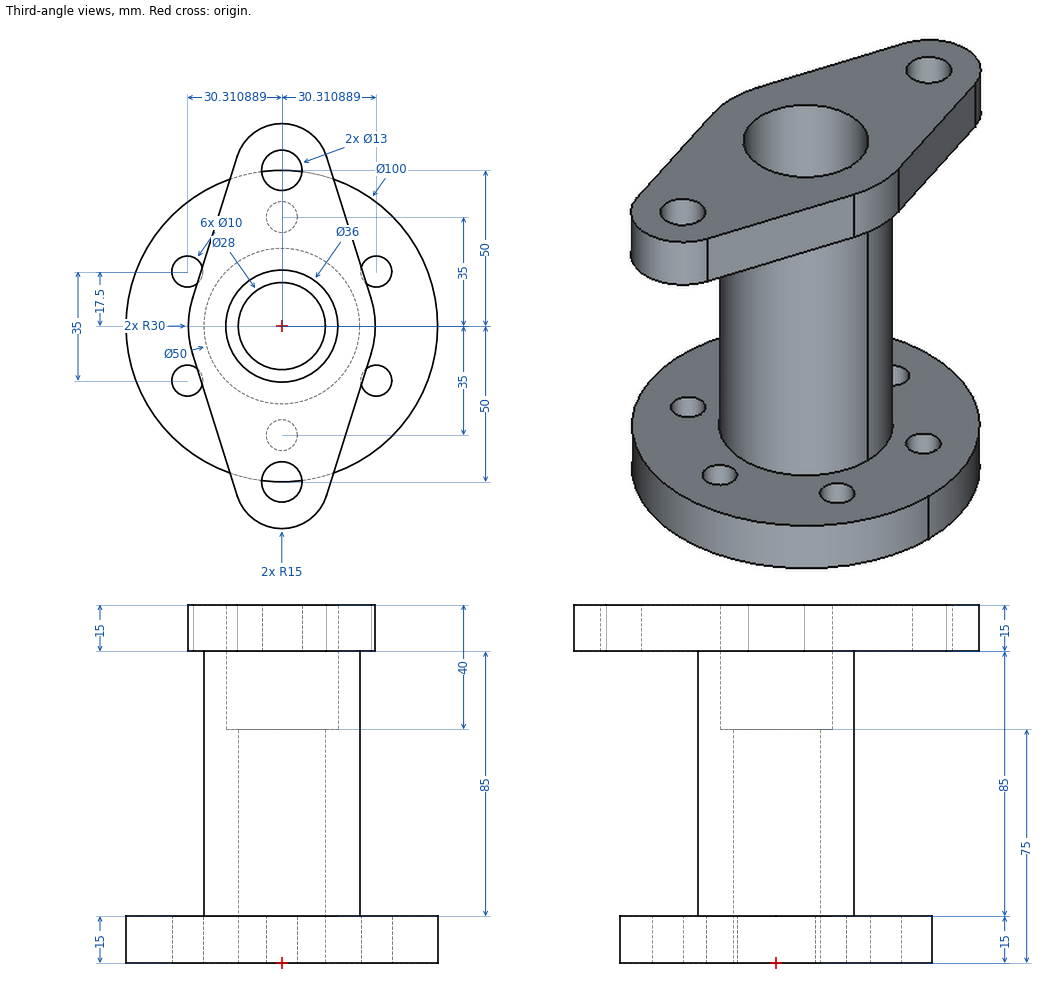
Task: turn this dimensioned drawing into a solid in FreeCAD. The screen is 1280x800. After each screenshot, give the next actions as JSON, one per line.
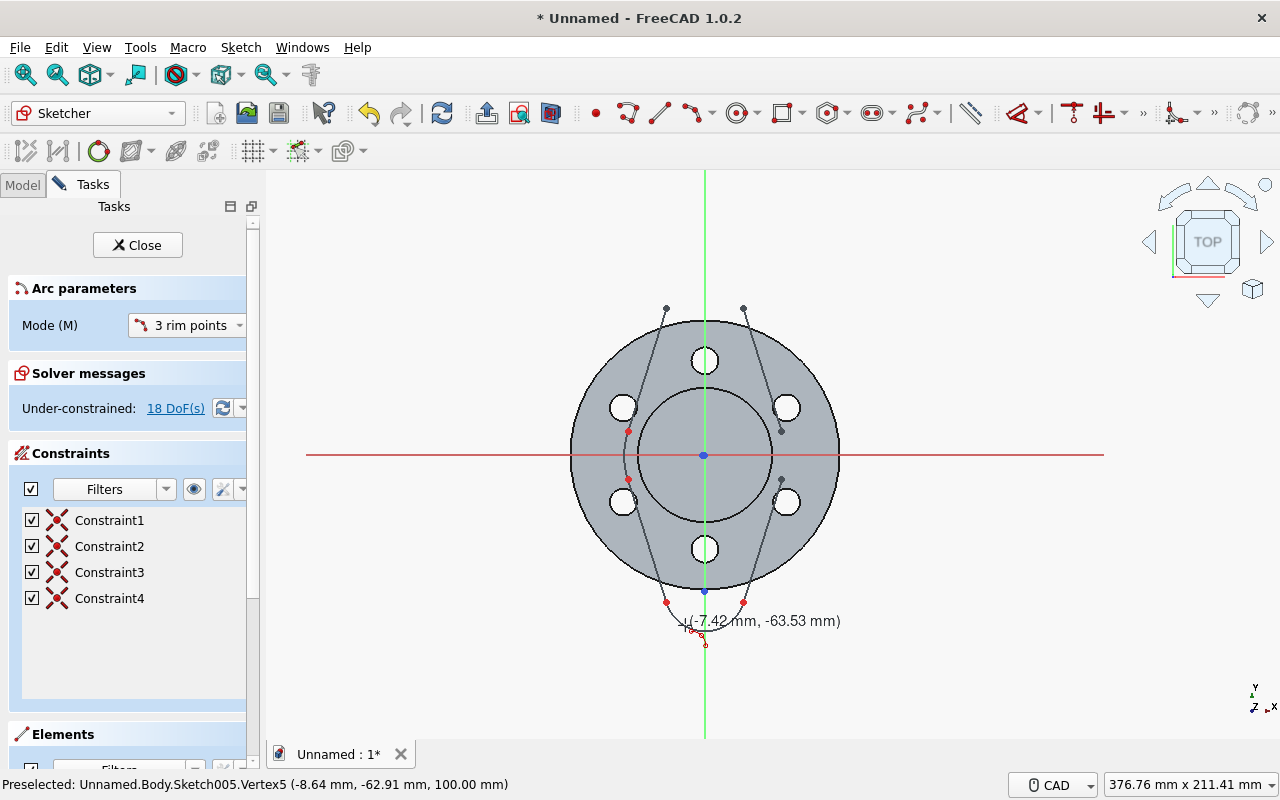
{"action": "left_click", "coordinate": [782, 480]}
{"action": "left_click", "coordinate": [782, 432]}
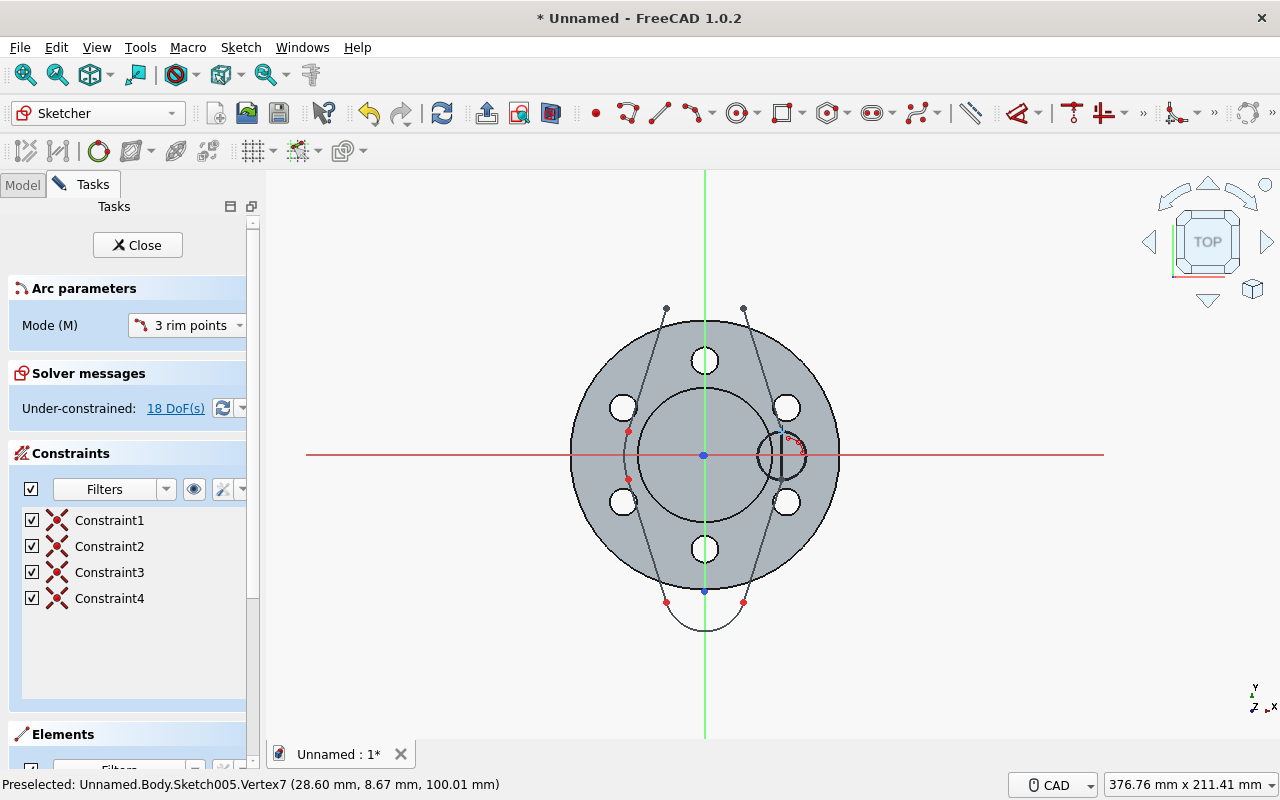
{"action": "scroll", "coordinate": [786, 460], "scroll_direction": "up", "scroll_amount": 8}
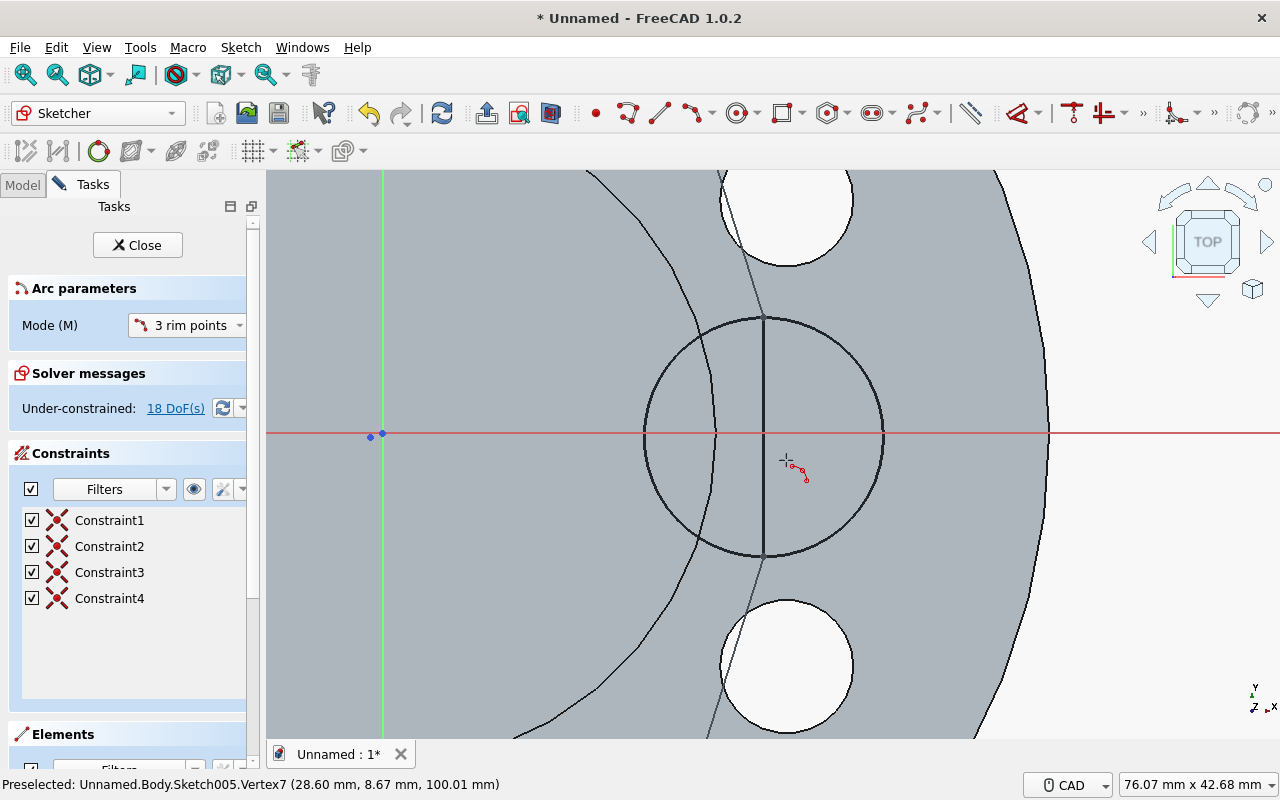
{"action": "left_click", "coordinate": [782, 458]}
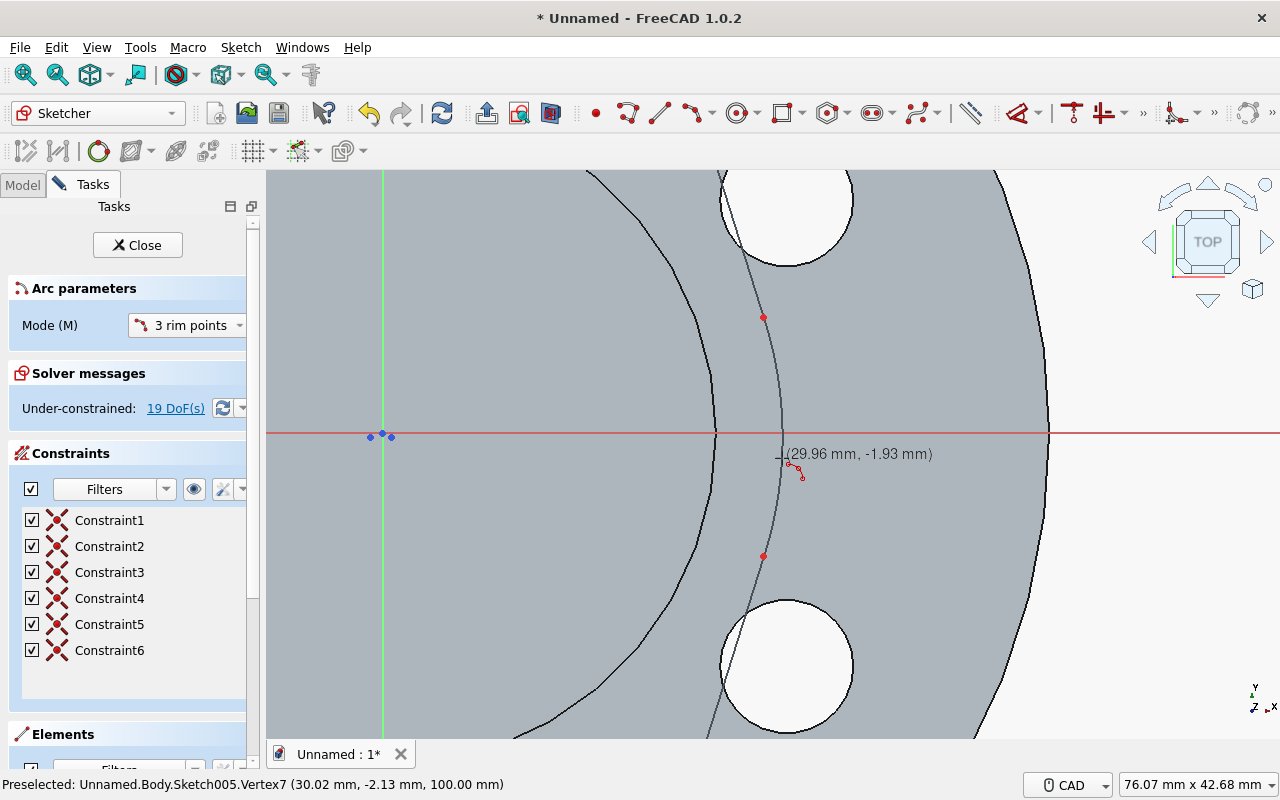
{"action": "scroll", "coordinate": [786, 460], "scroll_direction": "down", "scroll_amount": 8}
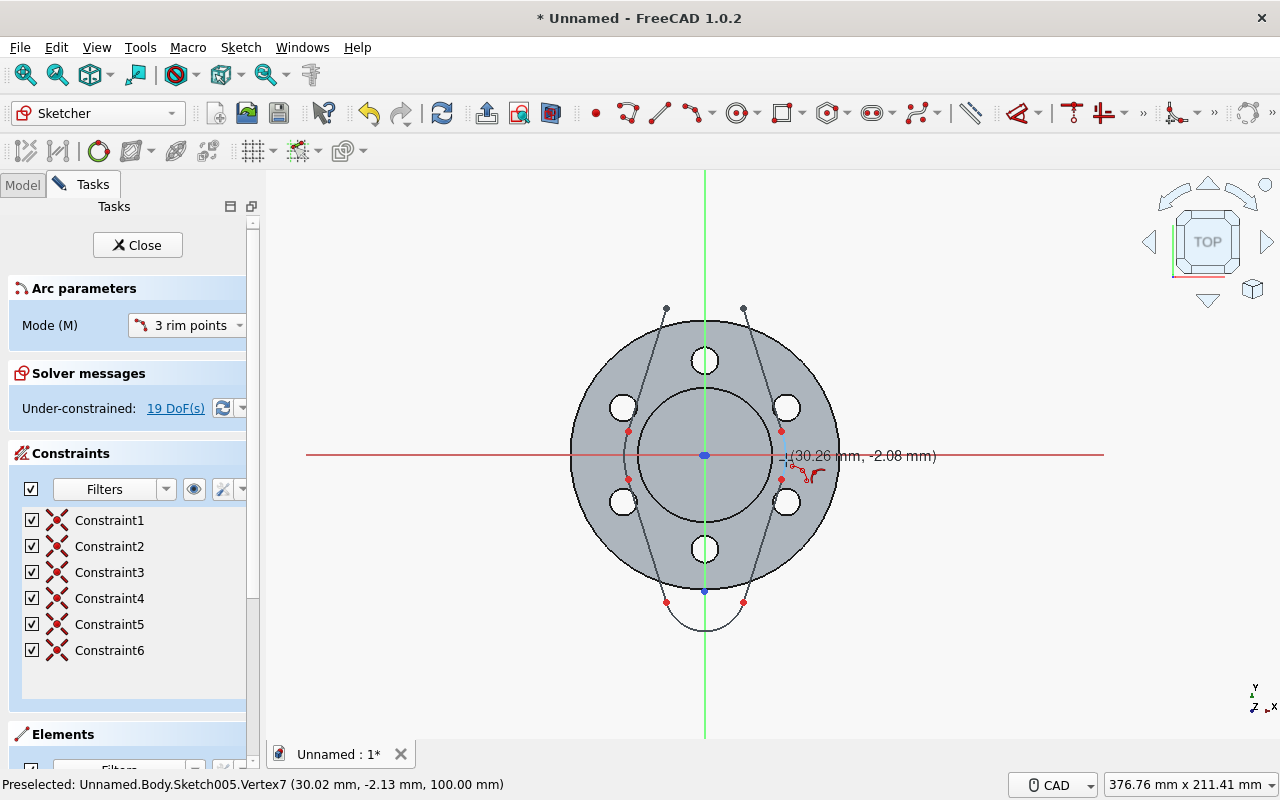
{"action": "left_click", "coordinate": [743, 309]}
{"action": "left_click", "coordinate": [666, 309]}
{"action": "left_click", "coordinate": [725, 285]}
{"action": "key", "text": "Escape"}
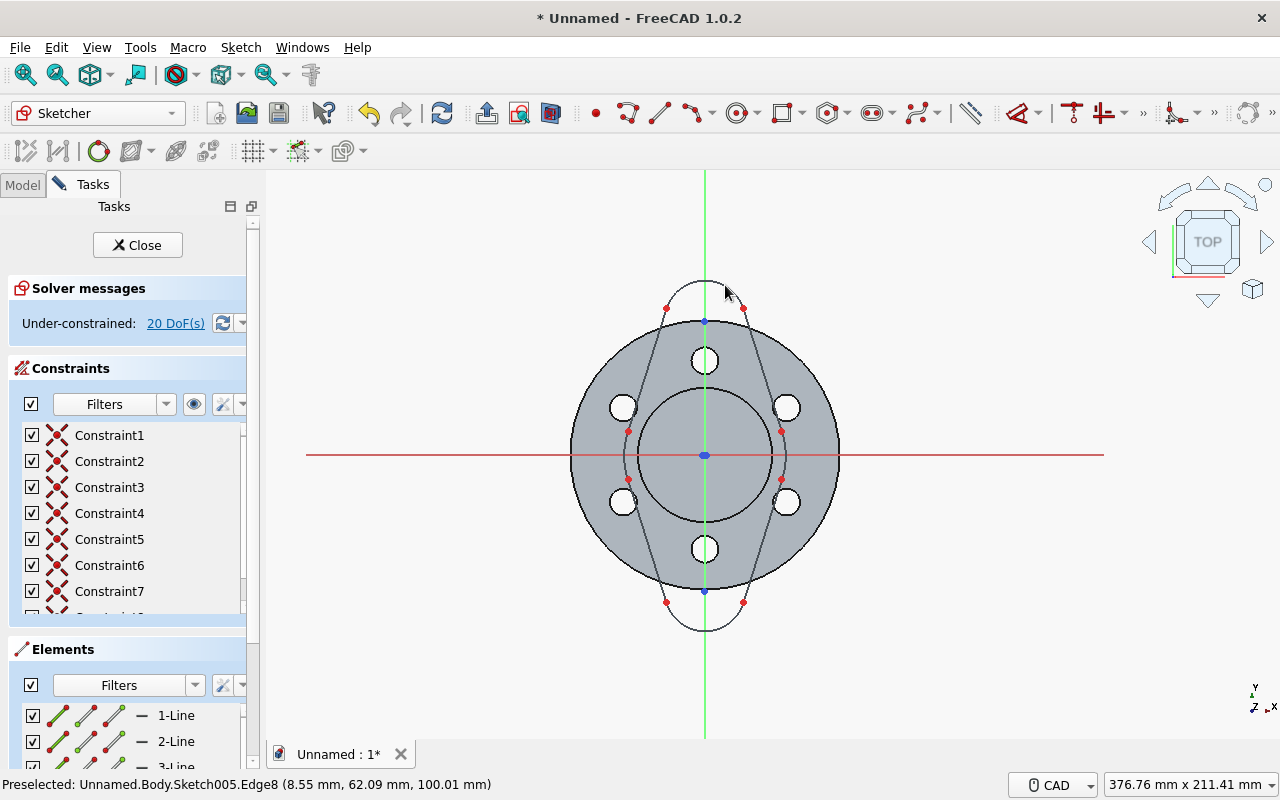
{"action": "left_click", "coordinate": [655, 346]}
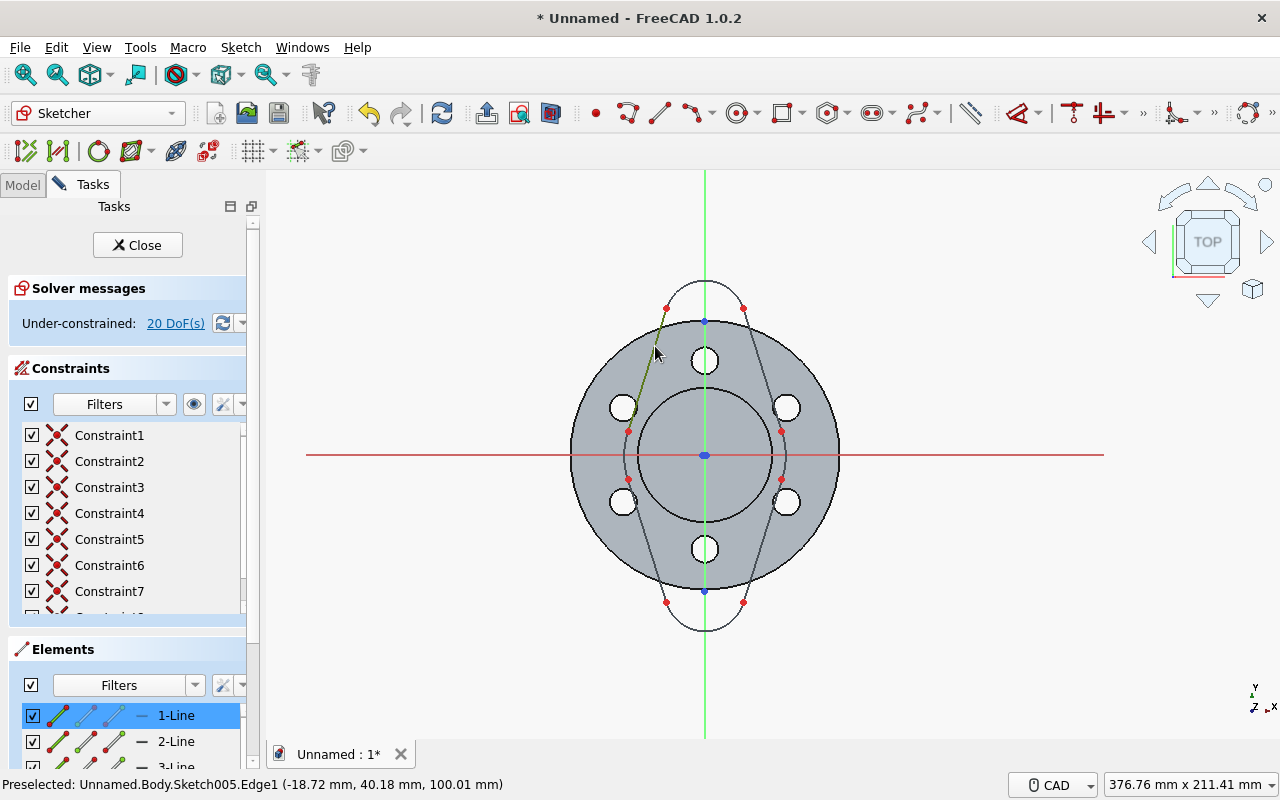
{"action": "scroll", "coordinate": [625, 466], "scroll_direction": "up", "scroll_amount": 2}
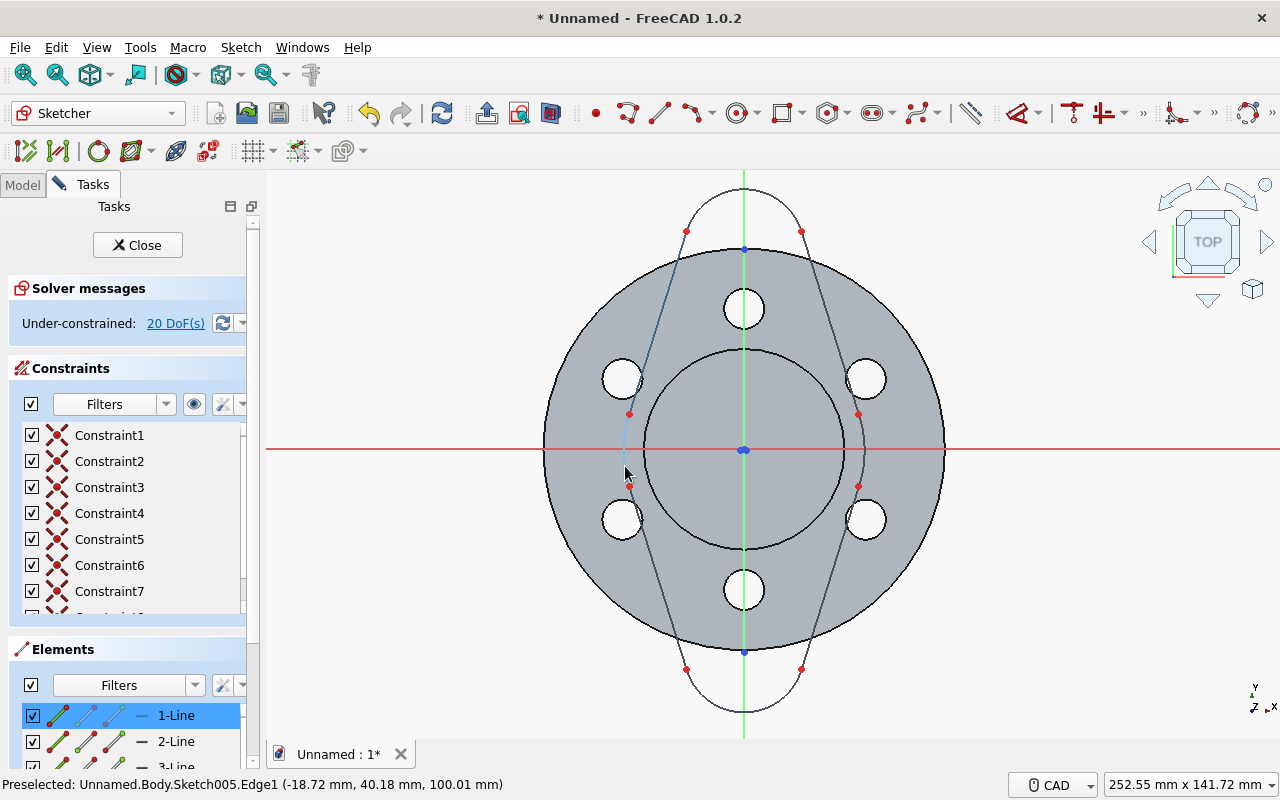
{"action": "left_click", "coordinate": [625, 465]}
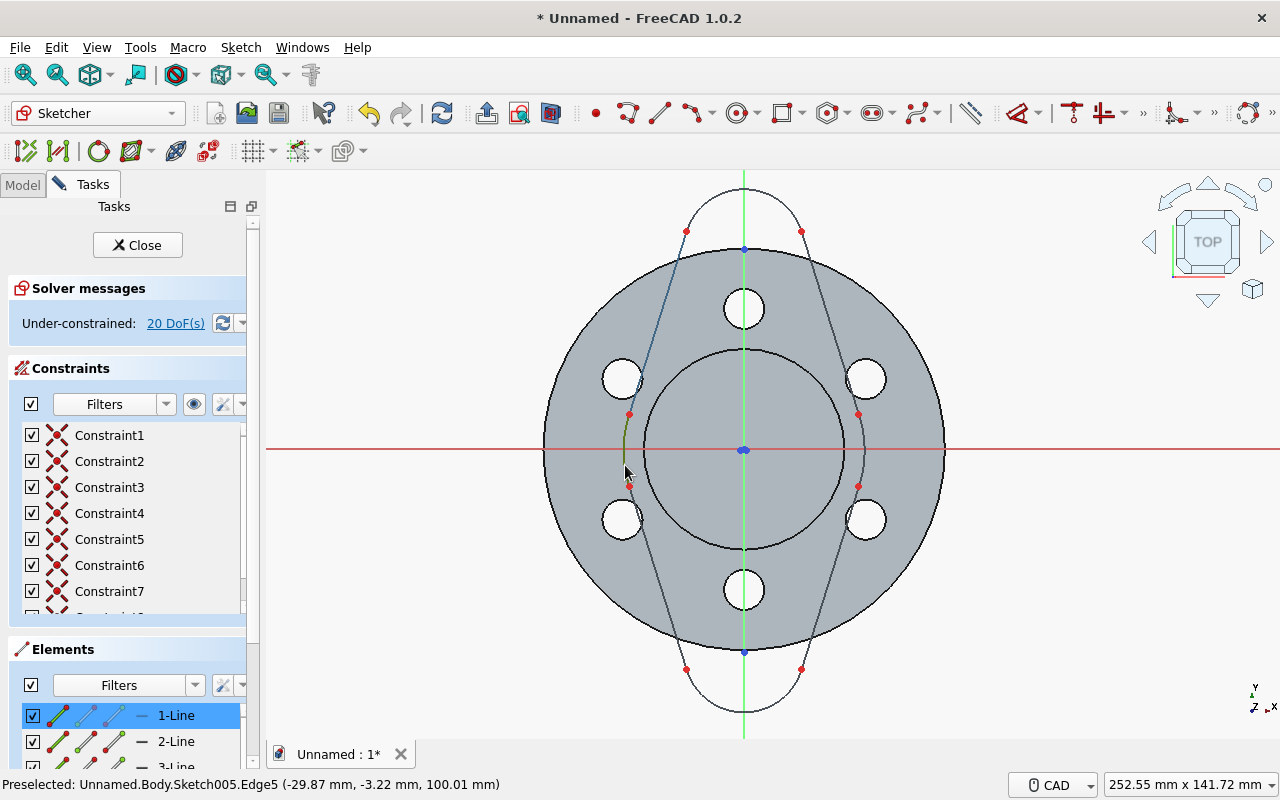
{"action": "key", "text": "t"}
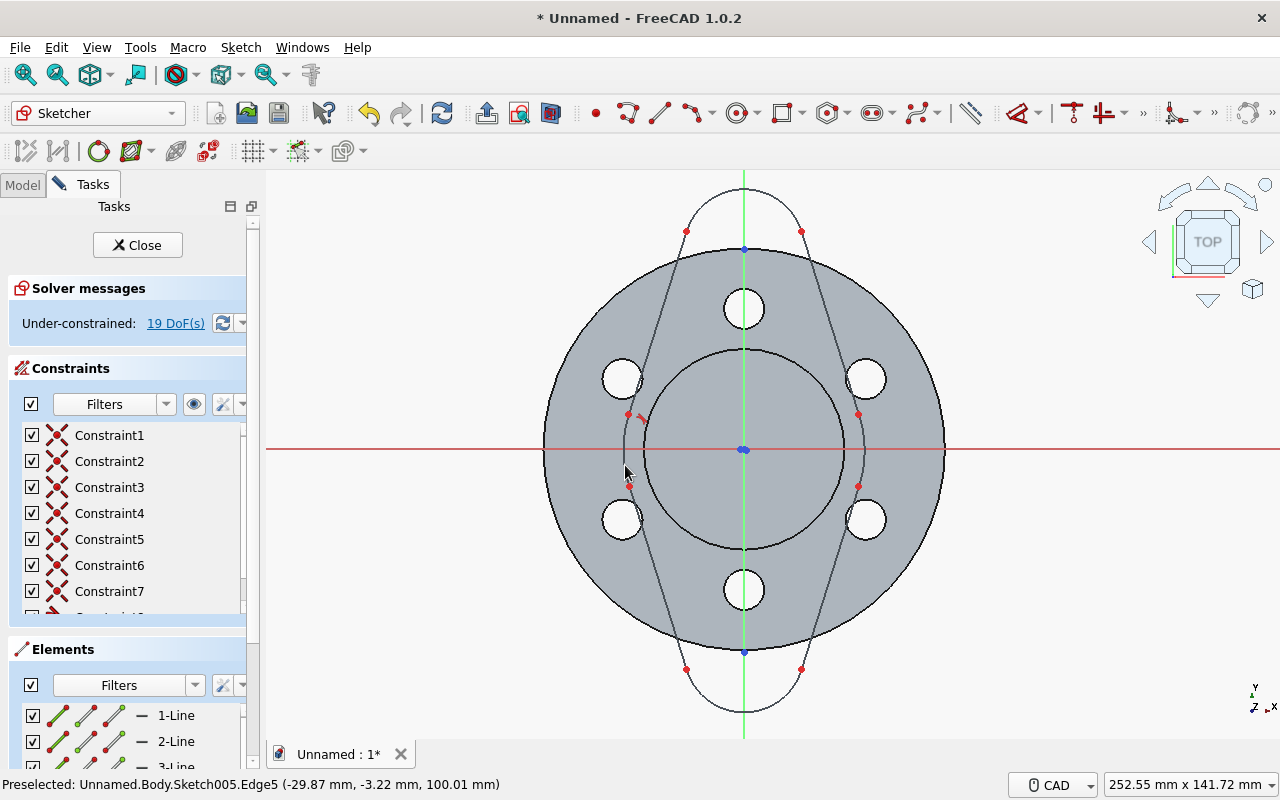
{"action": "left_click", "coordinate": [669, 286]}